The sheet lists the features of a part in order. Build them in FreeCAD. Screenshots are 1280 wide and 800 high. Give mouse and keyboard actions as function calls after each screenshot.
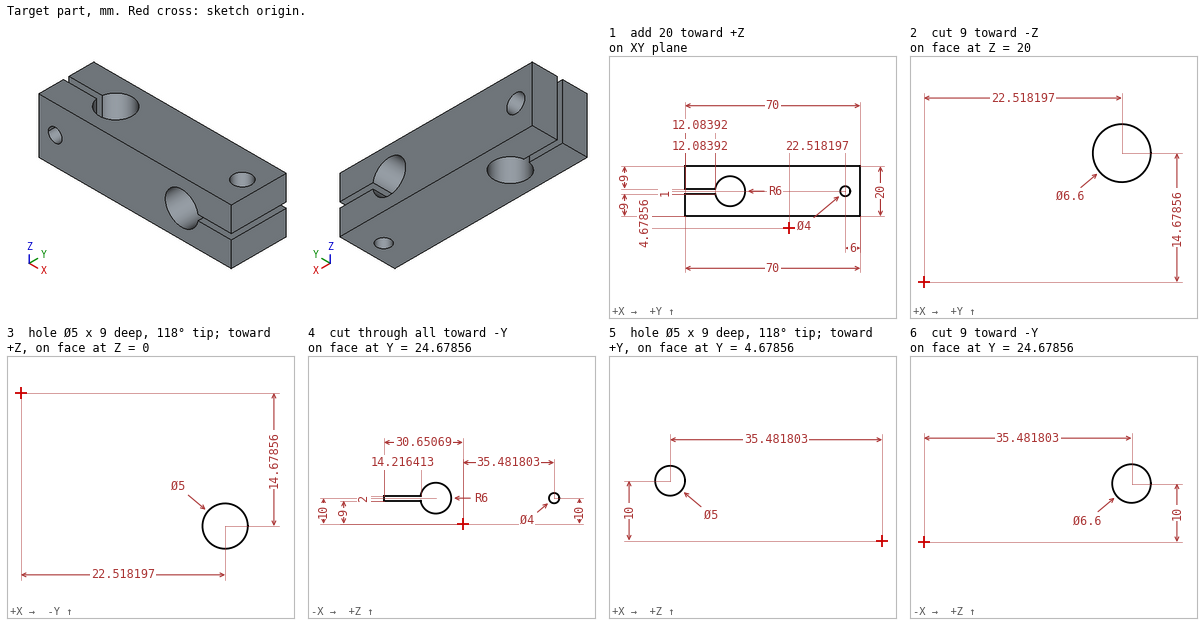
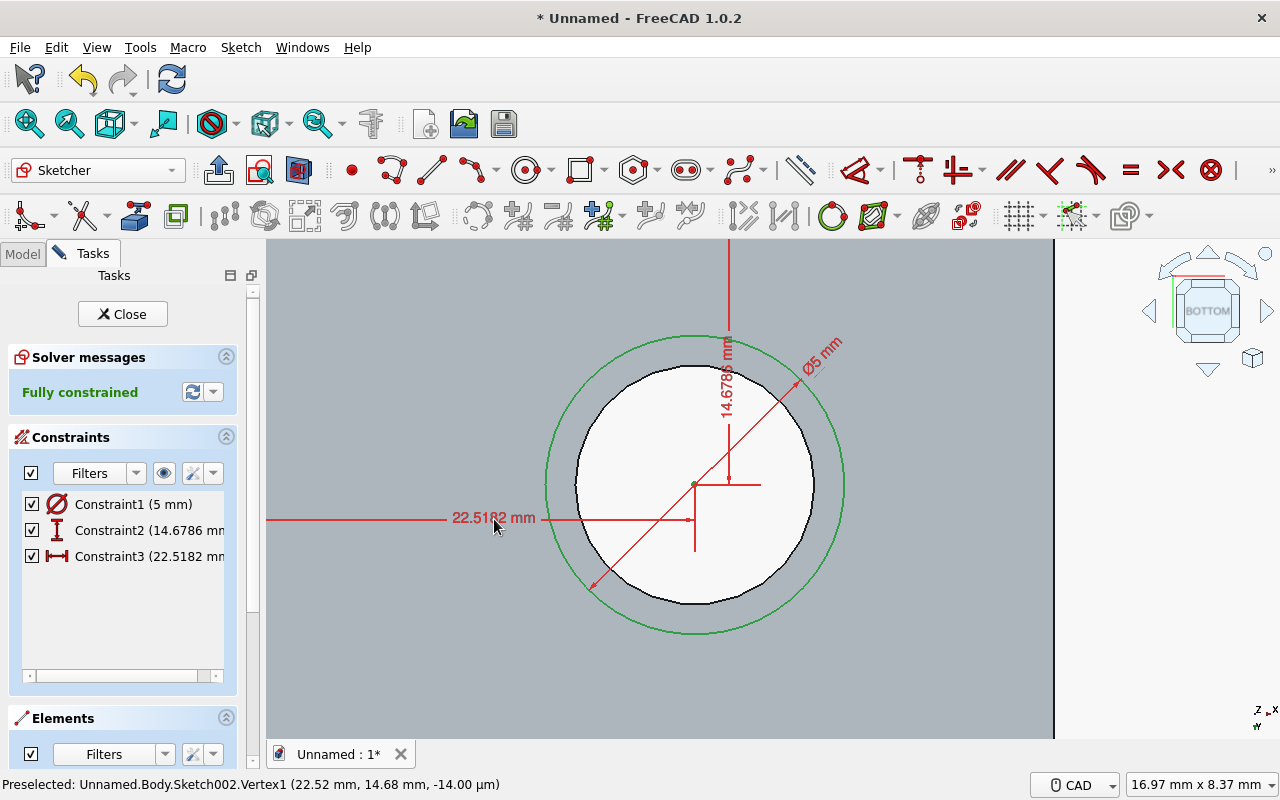
click(123, 314)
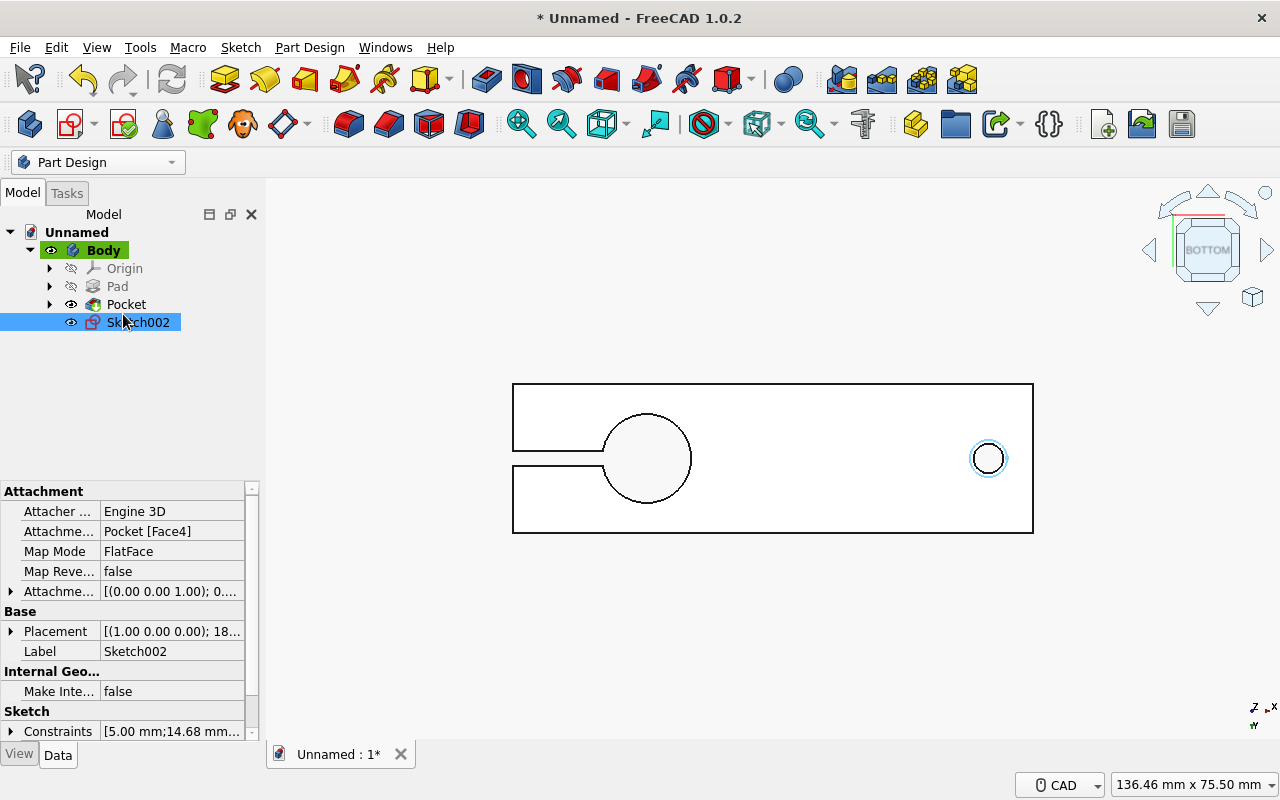
click(528, 80)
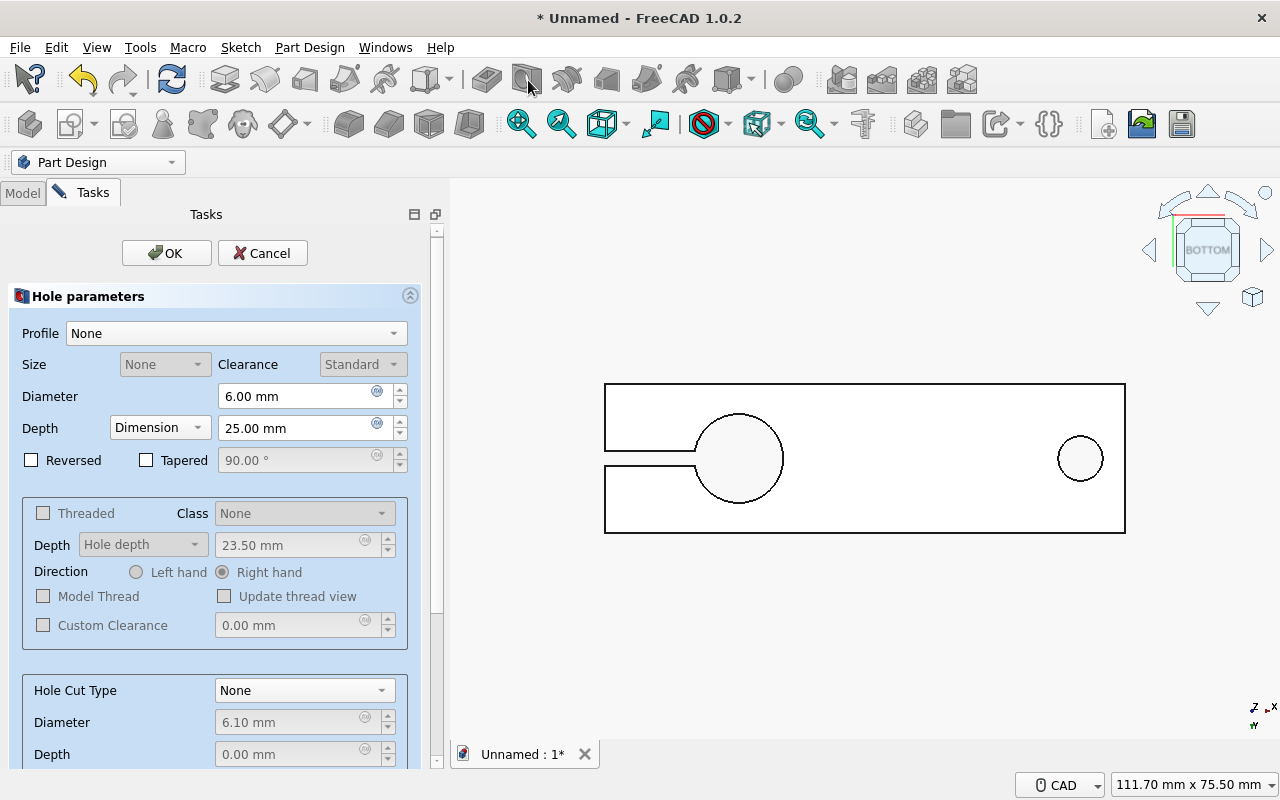
triple_click(305, 396)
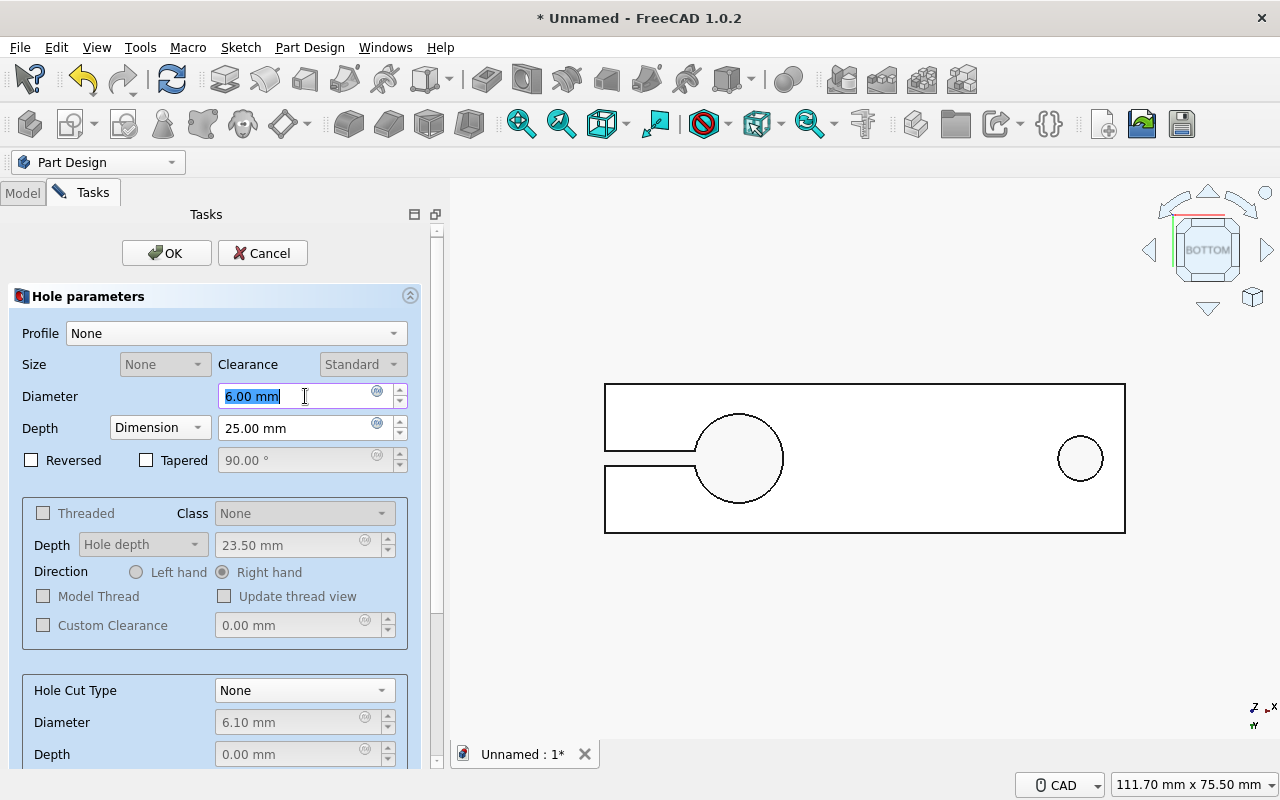
text(5)
key(Tab)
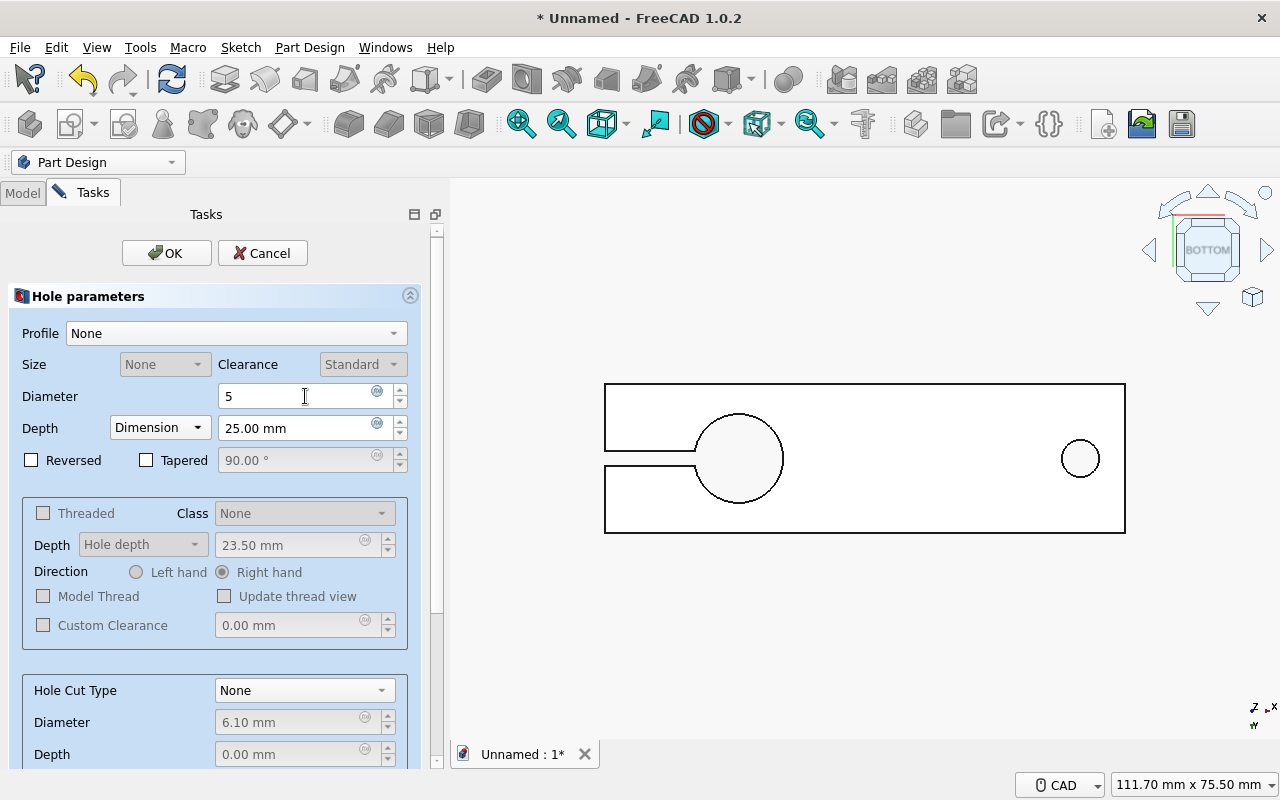
triple_click(305, 428)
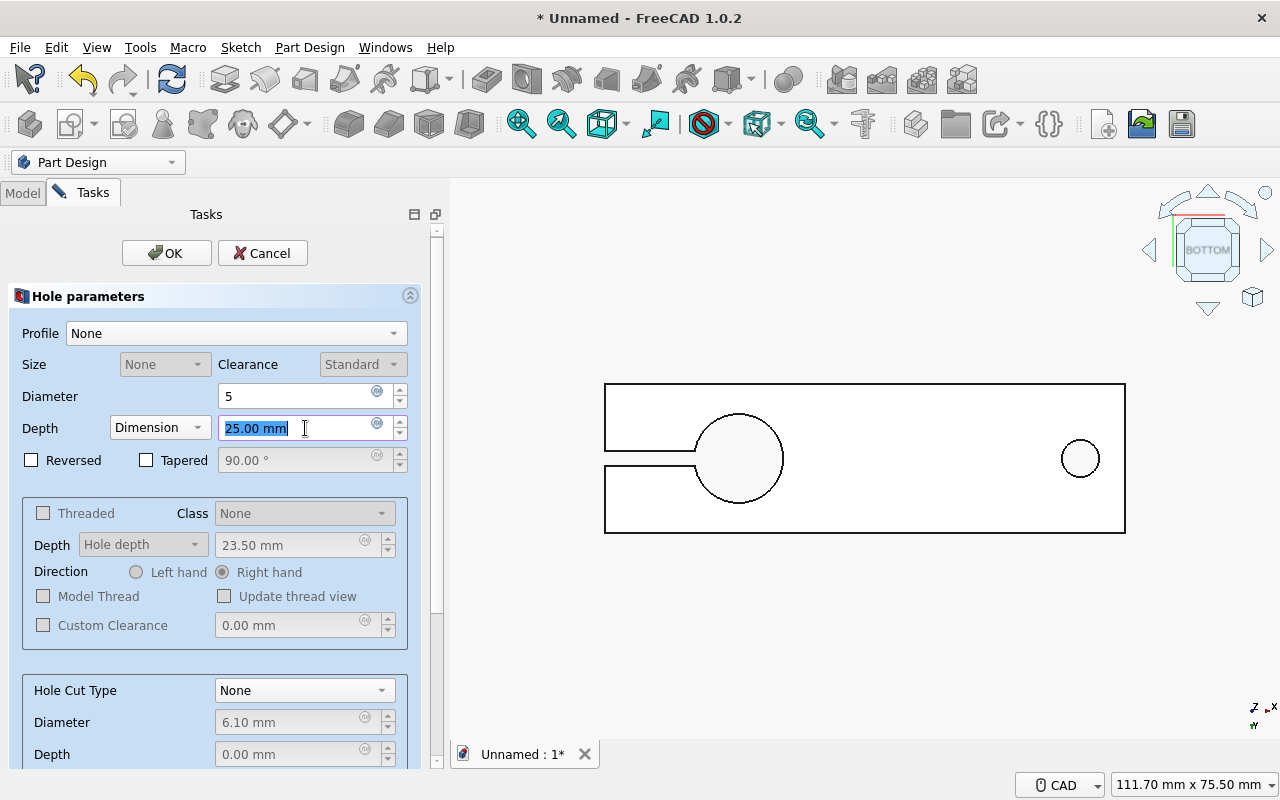
text(9)
key(Tab)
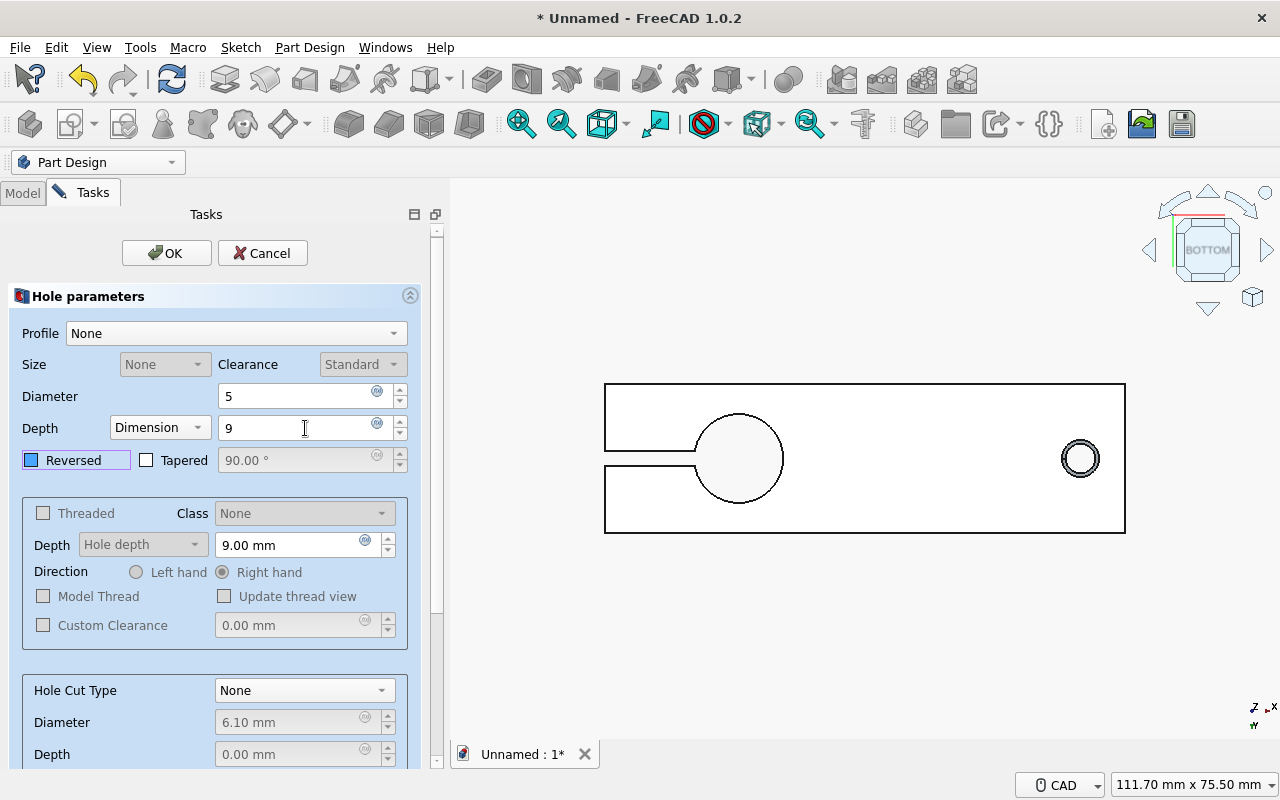
click(167, 253)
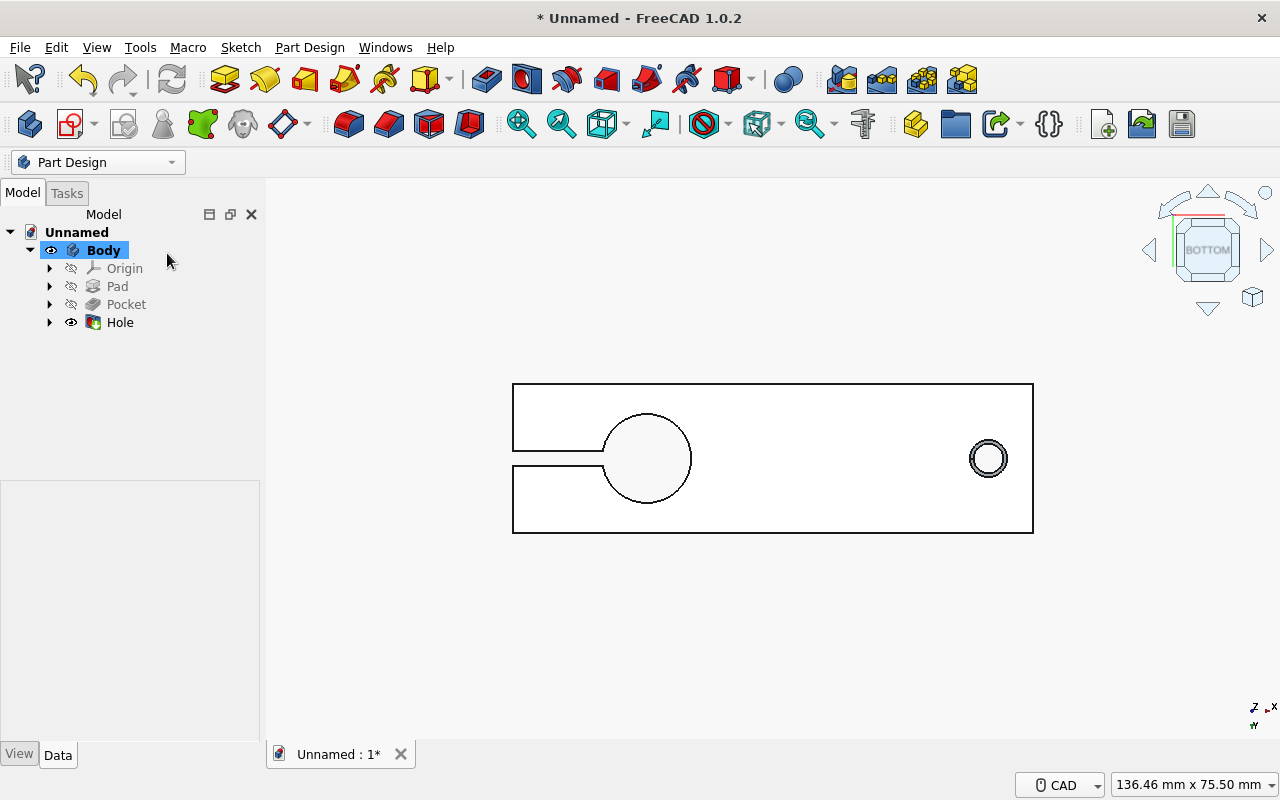
key(4)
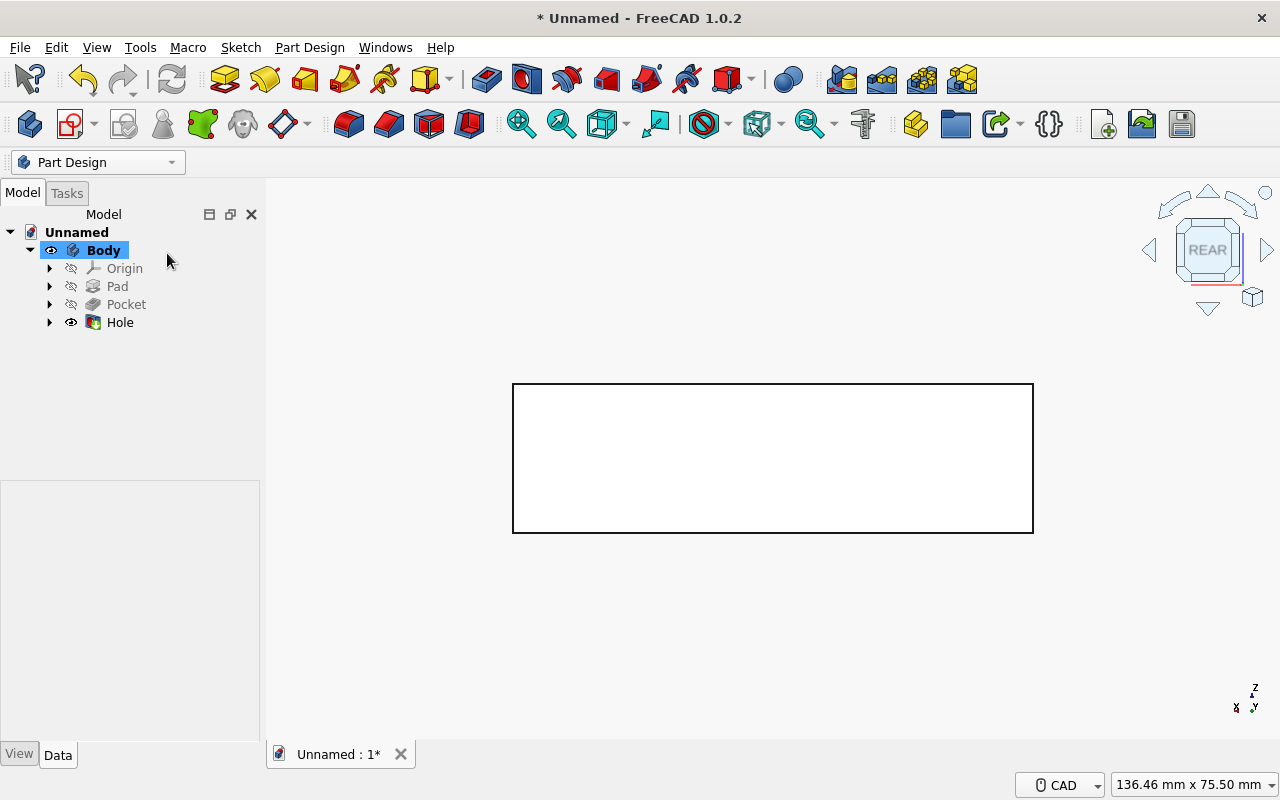
click(624, 457)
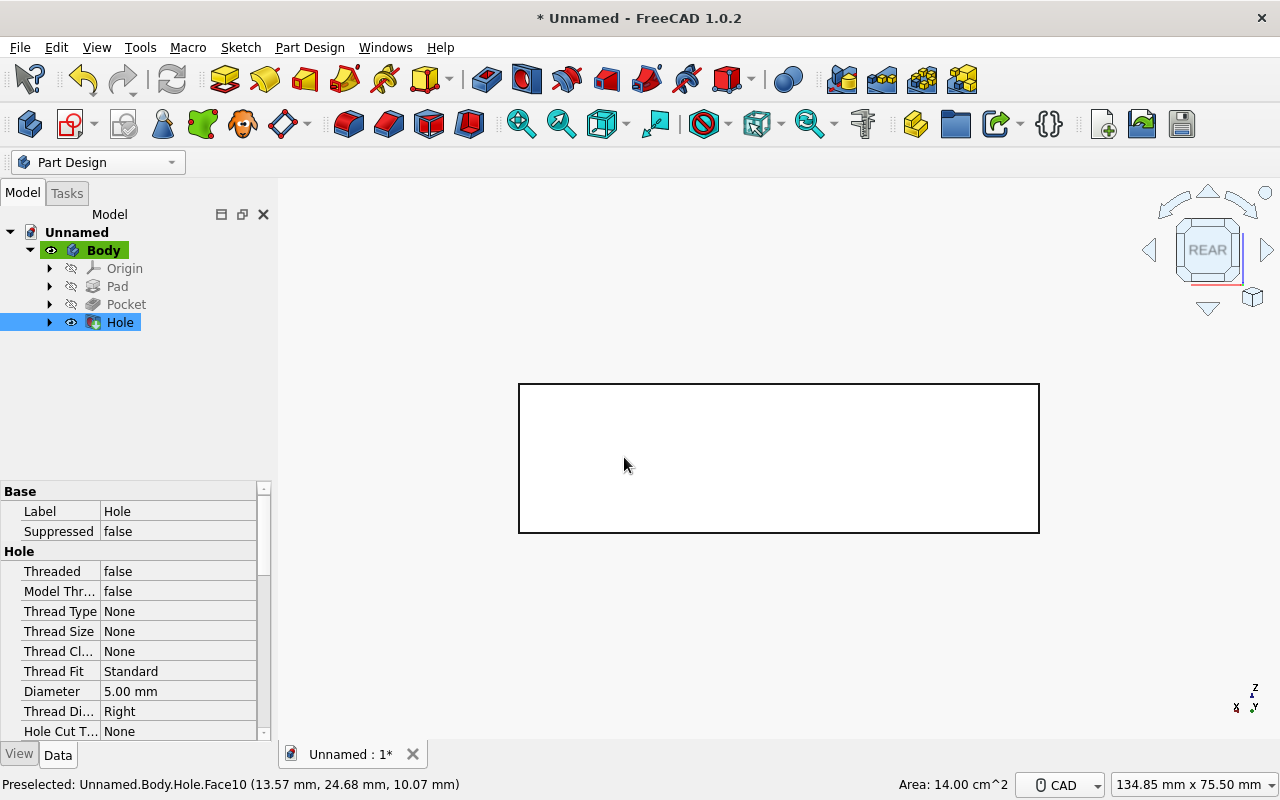
click(70, 124)